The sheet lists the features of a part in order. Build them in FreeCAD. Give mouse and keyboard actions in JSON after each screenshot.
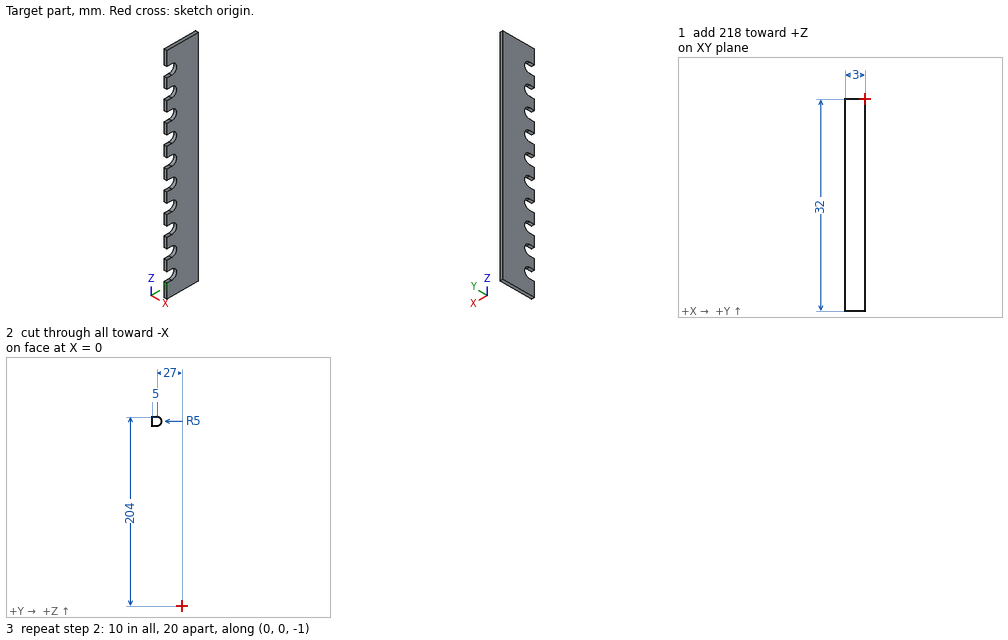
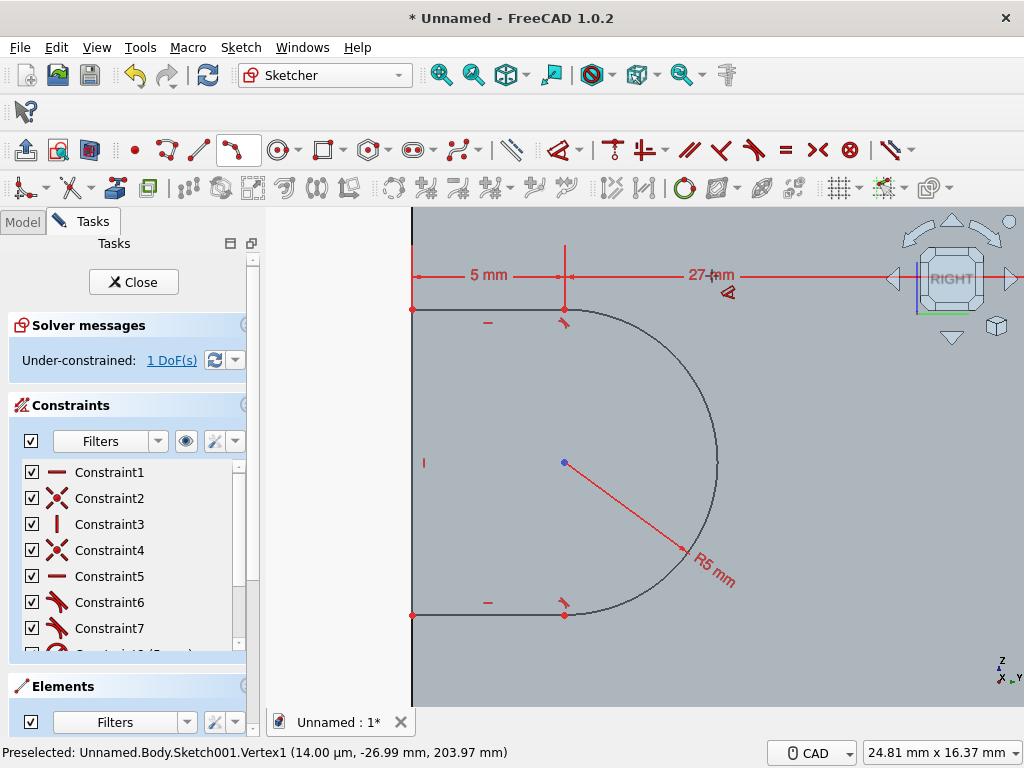
{"action": "left_click", "coordinate": [565, 310]}
{"action": "left_click", "coordinate": [531, 494]}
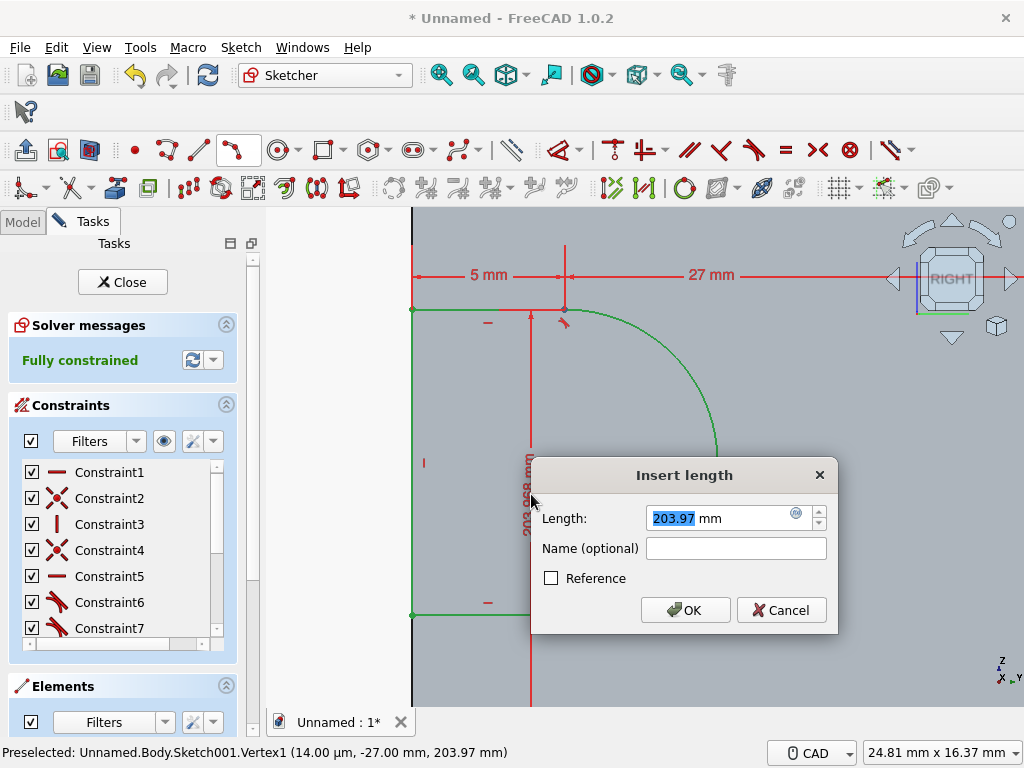
{"action": "type", "text": "204"}
{"action": "key", "text": "Return"}
{"action": "key", "text": "Escape"}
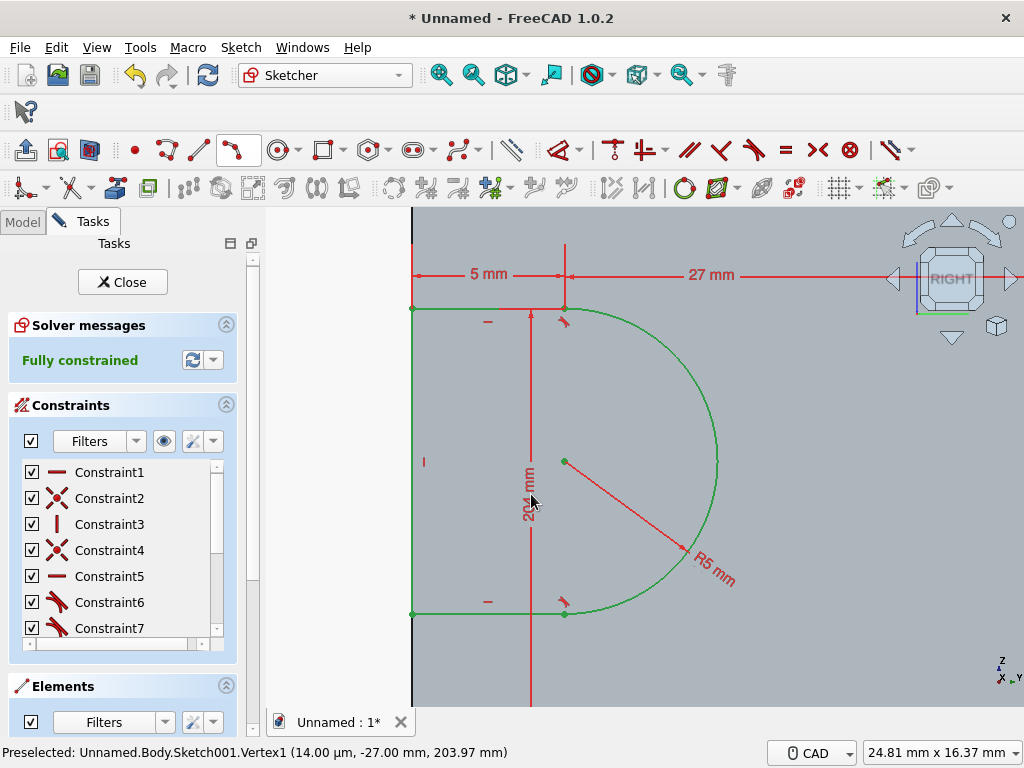
{"action": "left_click", "coordinate": [123, 282]}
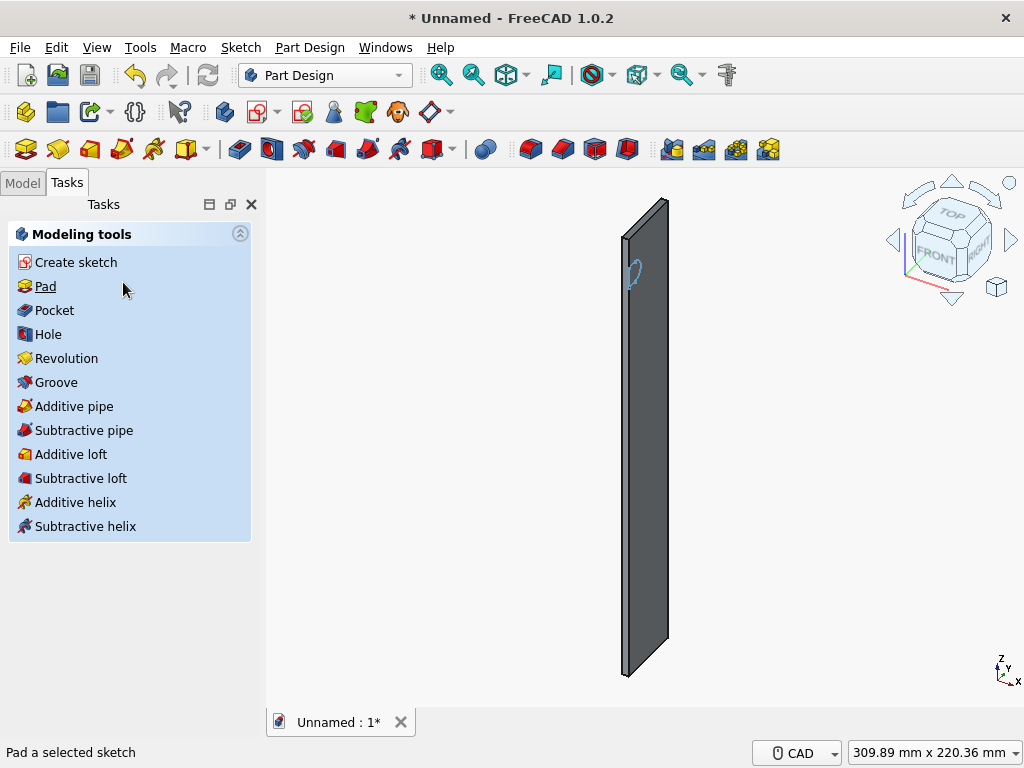
{"action": "left_click", "coordinate": [240, 150]}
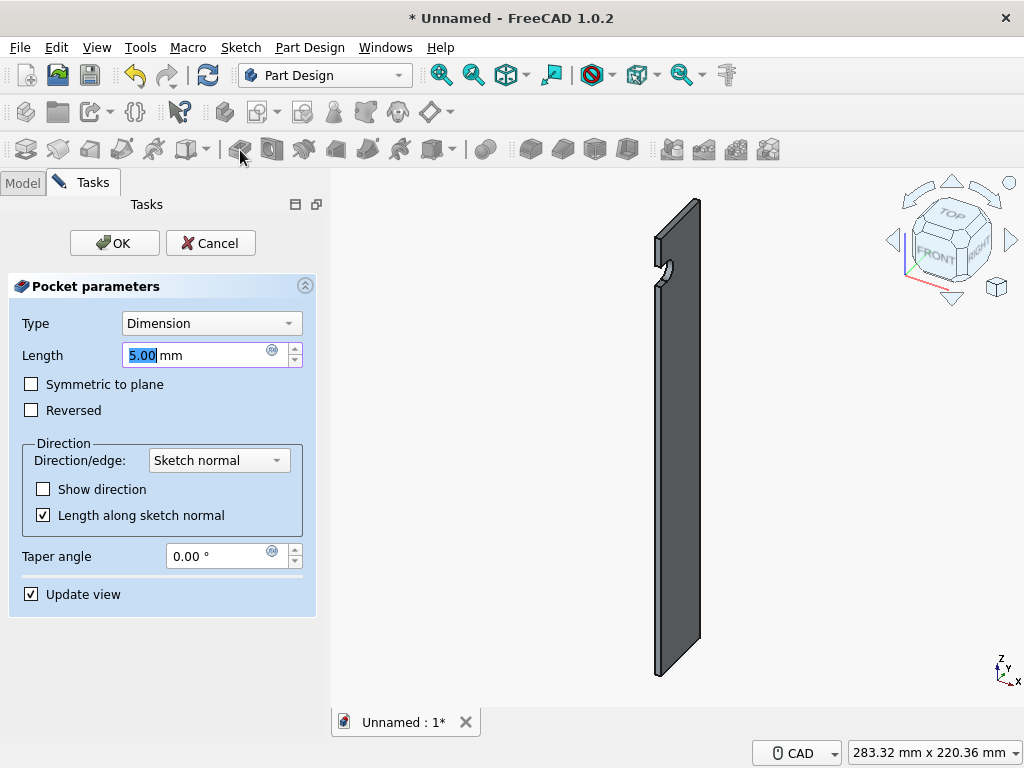
{"action": "left_click", "coordinate": [212, 324]}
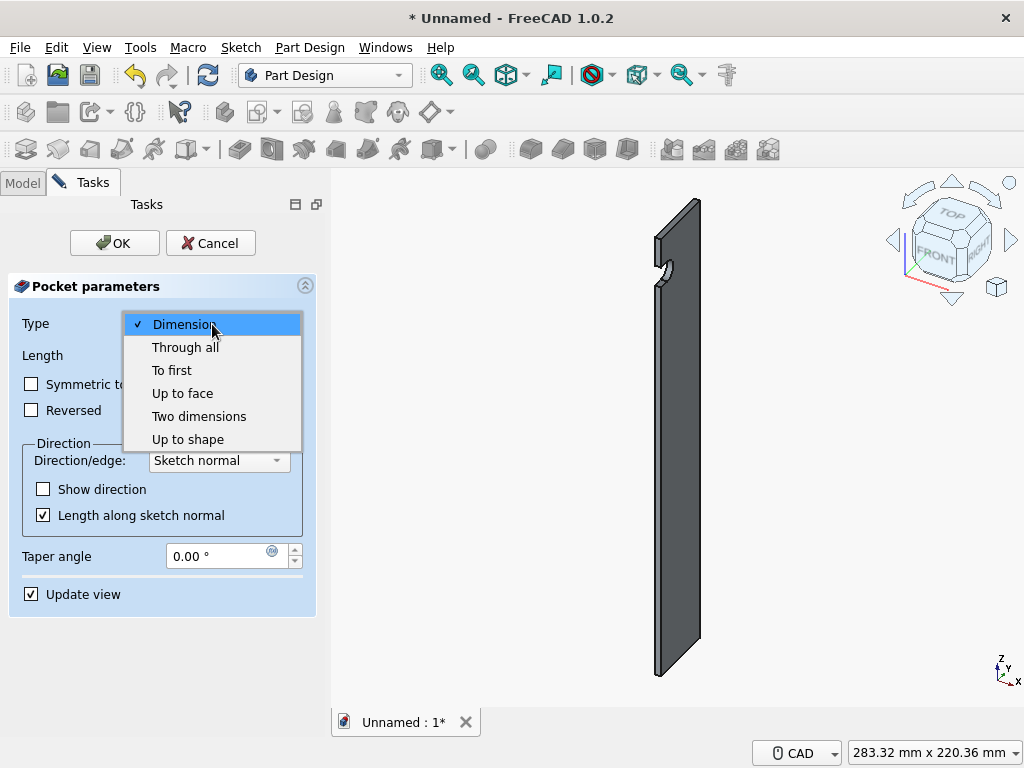
{"action": "left_click", "coordinate": [212, 348]}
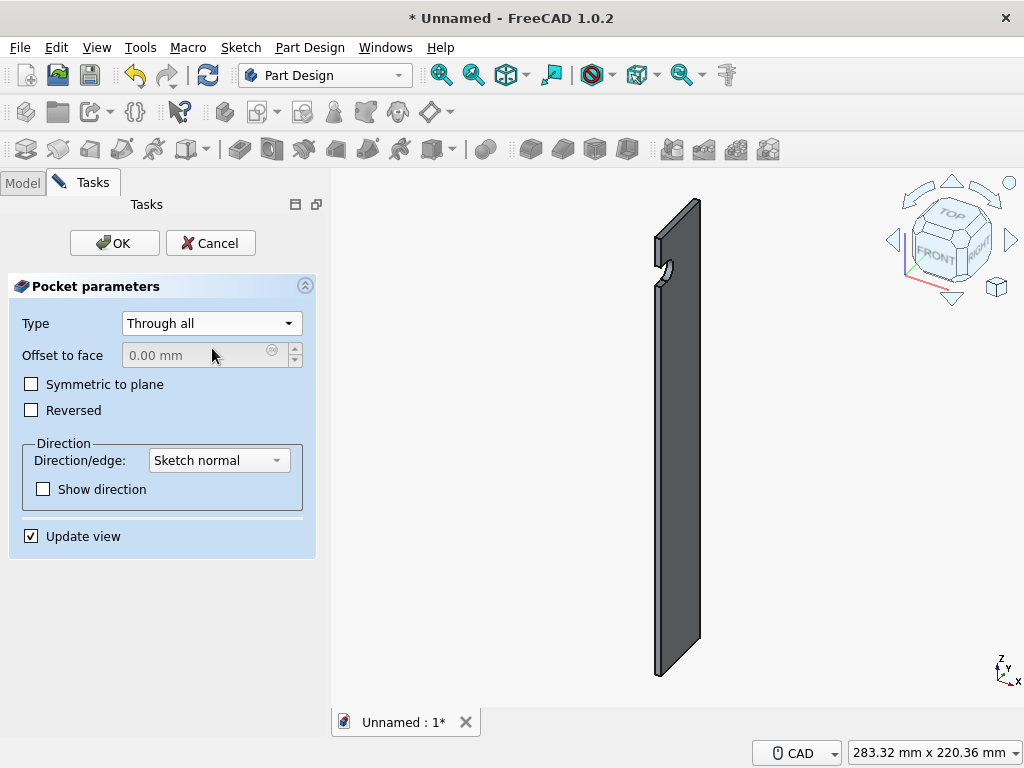
{"action": "left_click", "coordinate": [115, 243]}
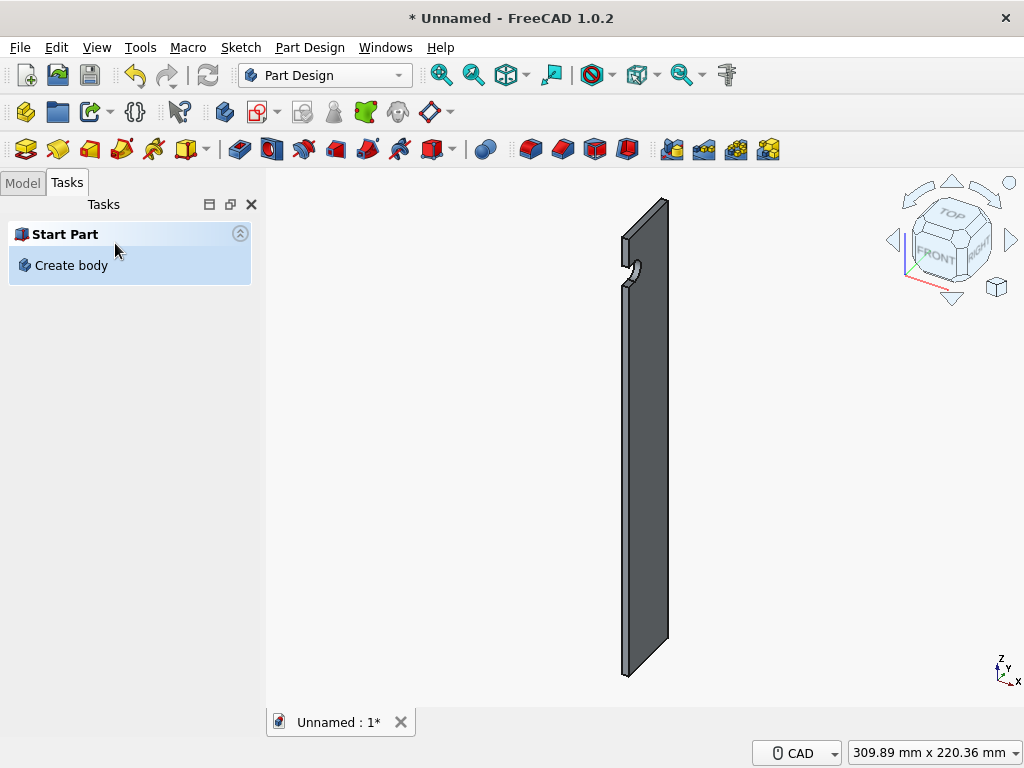
{"action": "left_click", "coordinate": [23, 182]}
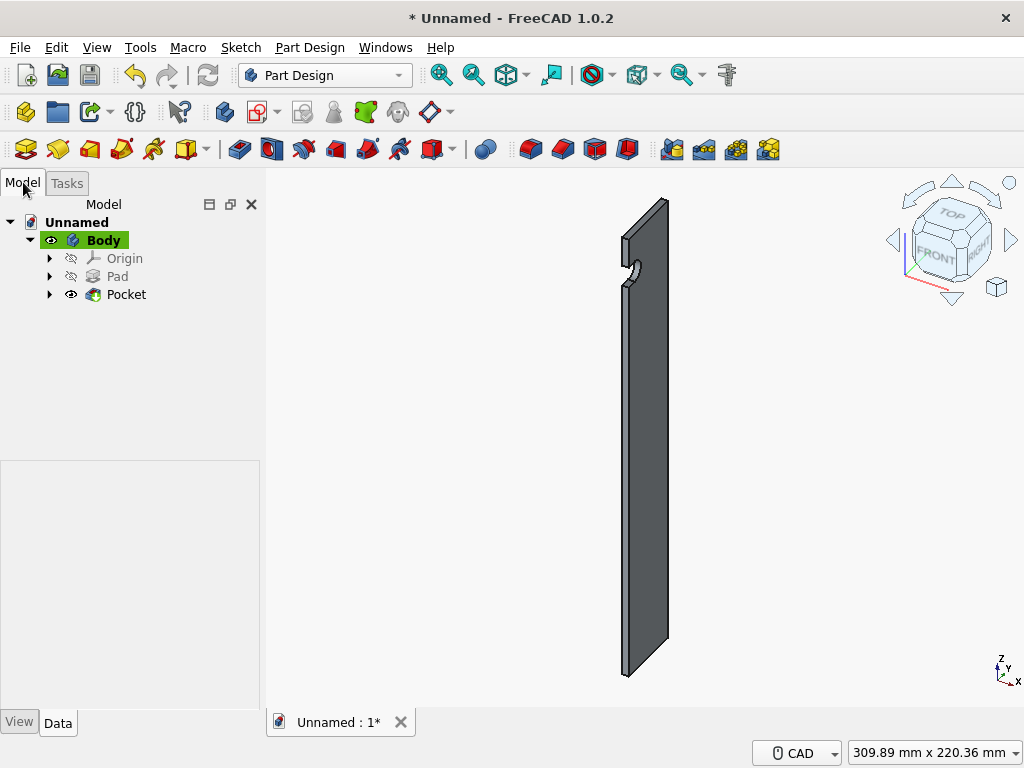
{"action": "left_click", "coordinate": [116, 294]}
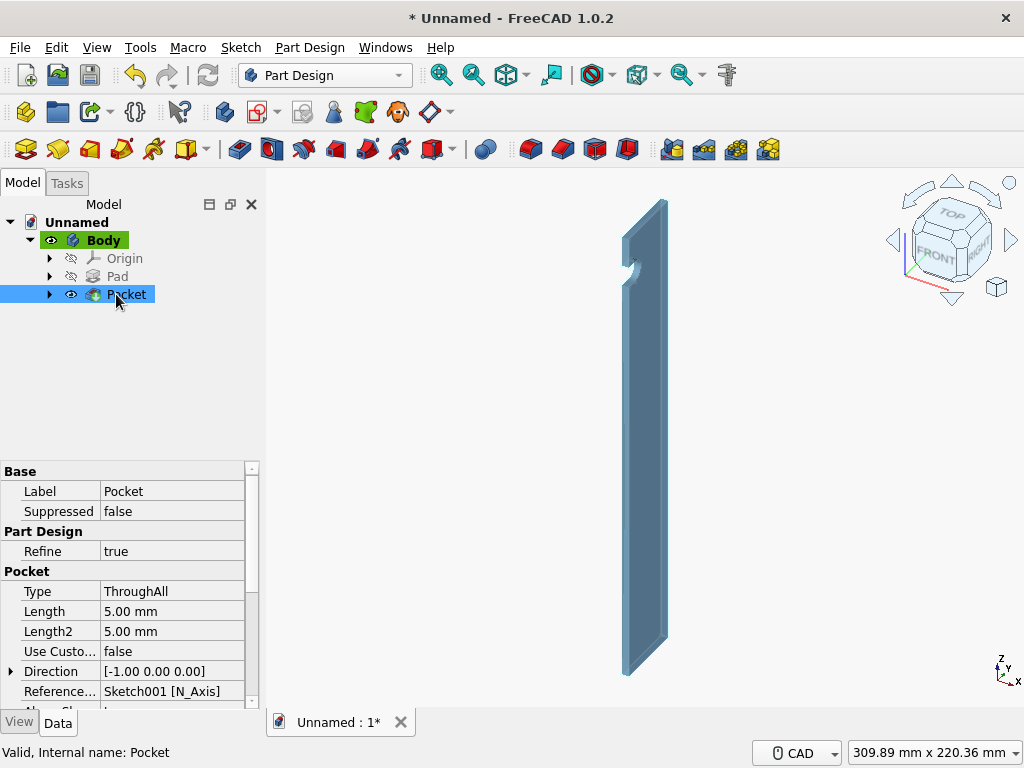
{"action": "left_click", "coordinate": [704, 150]}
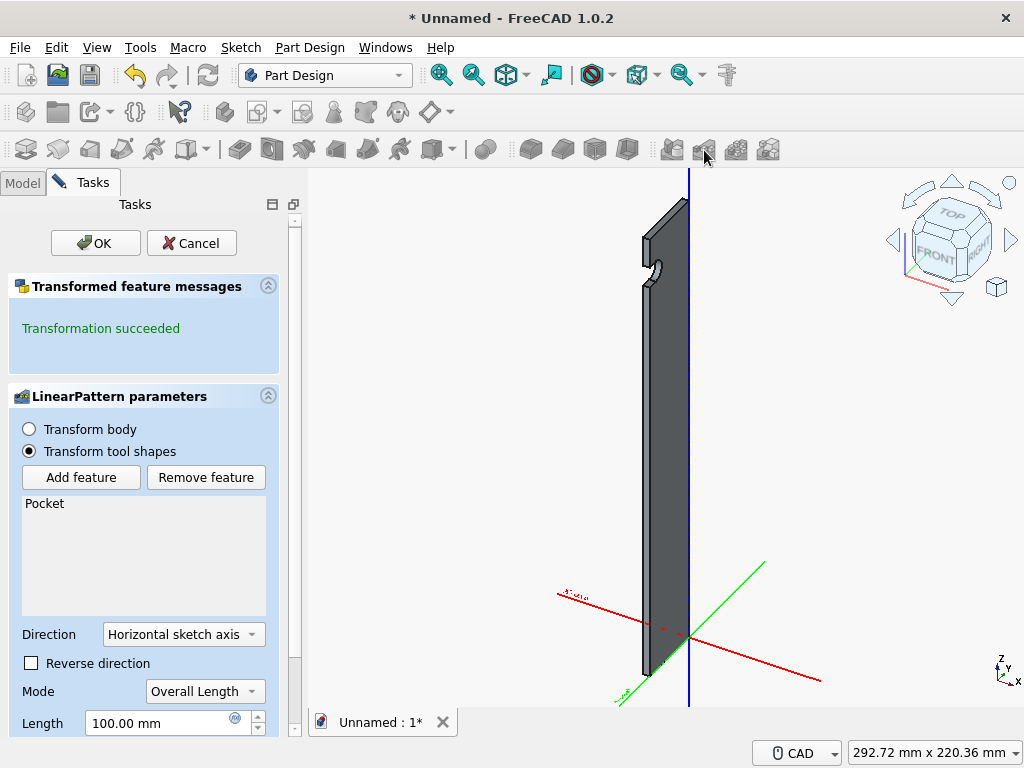
{"action": "left_click", "coordinate": [184, 634]}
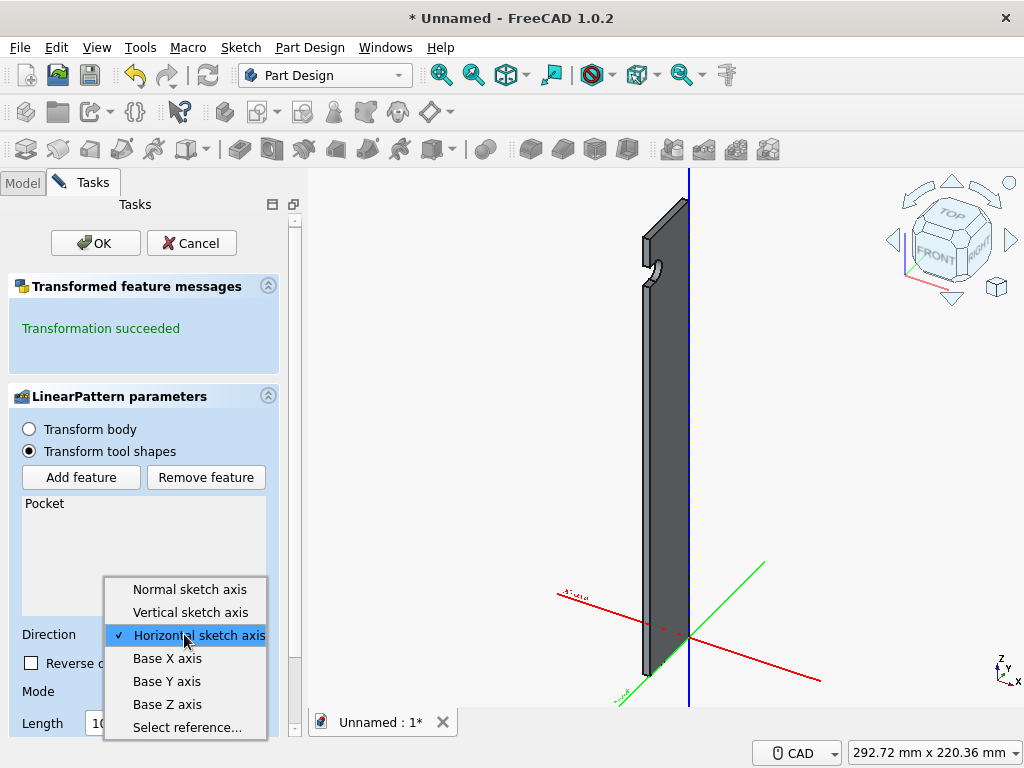
{"action": "left_click", "coordinate": [184, 704]}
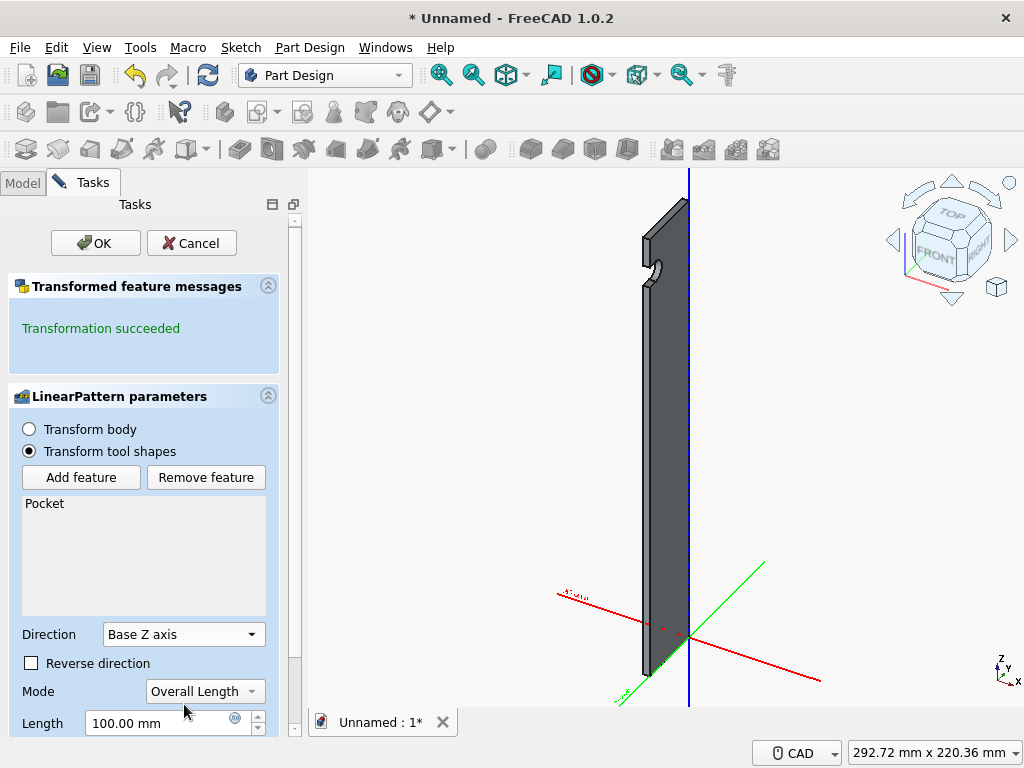
{"action": "left_click", "coordinate": [206, 692]}